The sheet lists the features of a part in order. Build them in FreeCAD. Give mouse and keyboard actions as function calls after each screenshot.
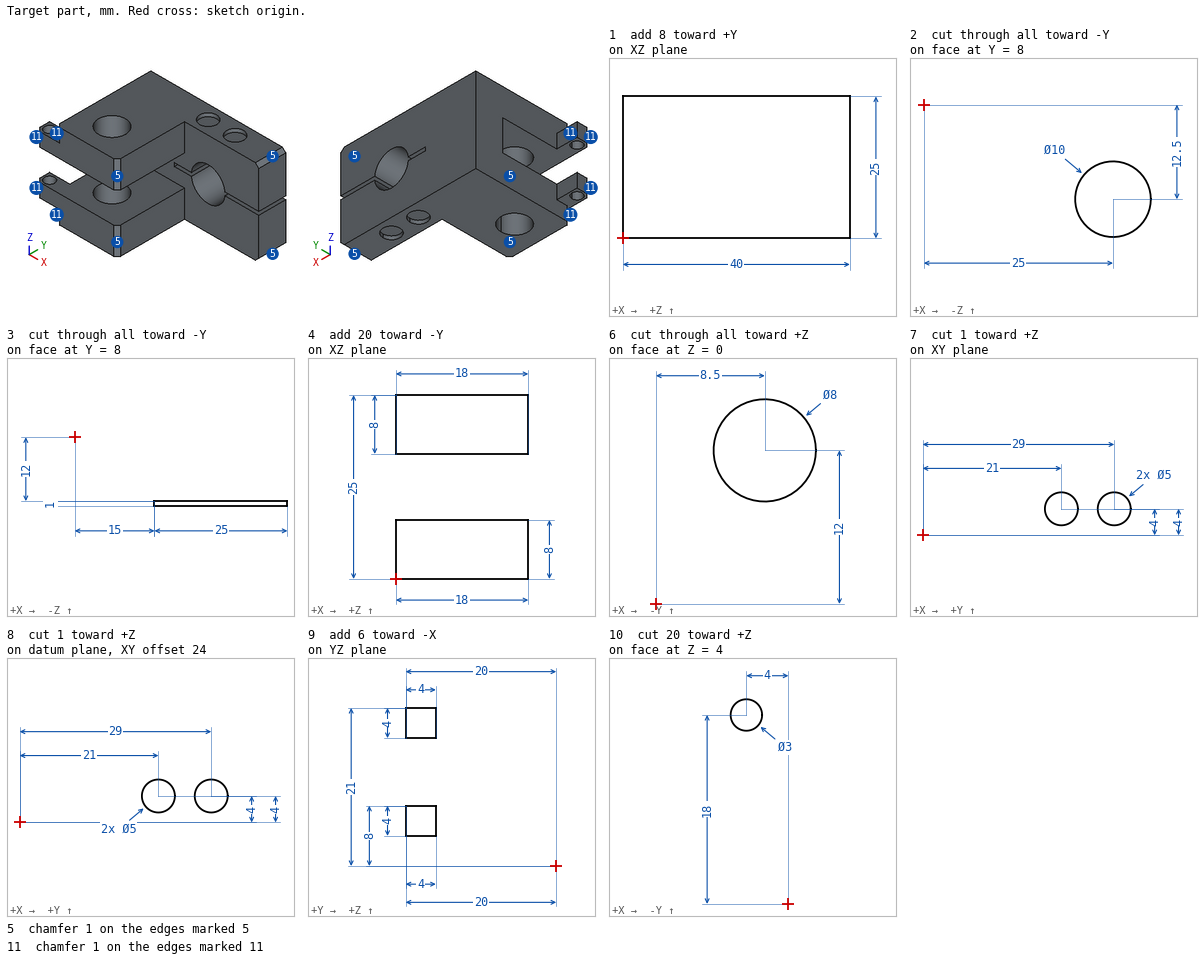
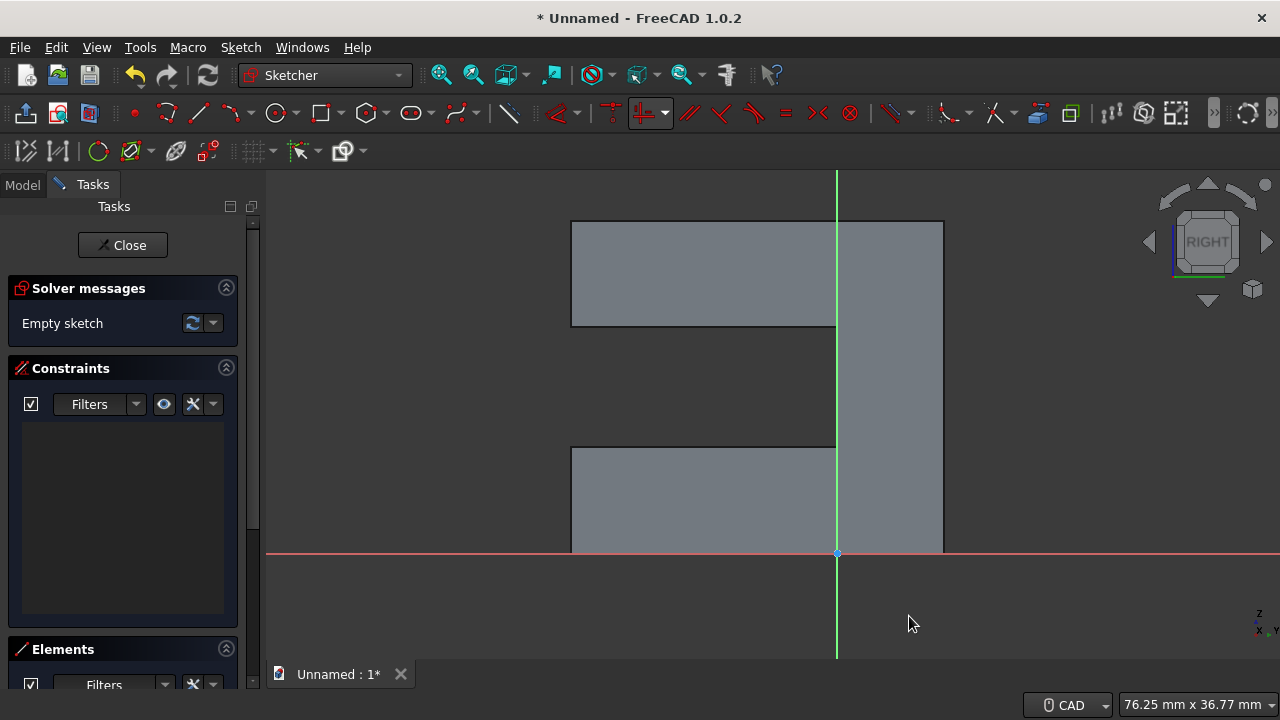
click(322, 114)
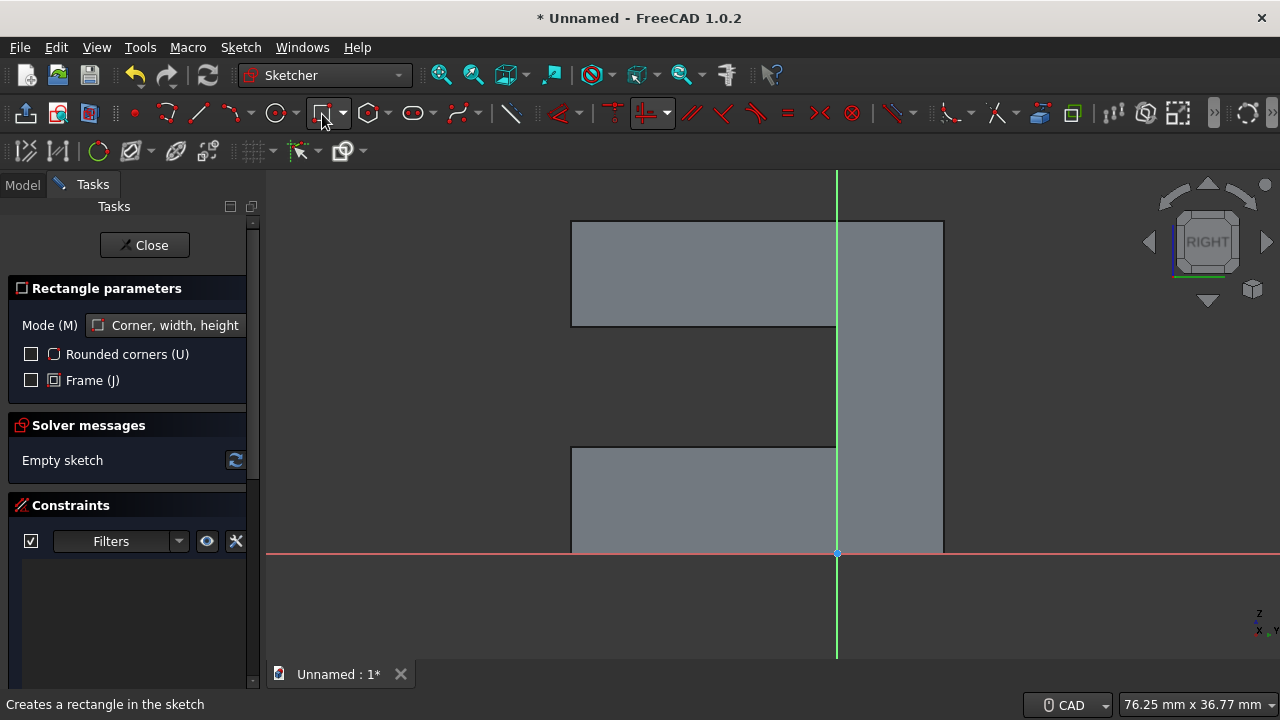
click(571, 274)
click(624, 327)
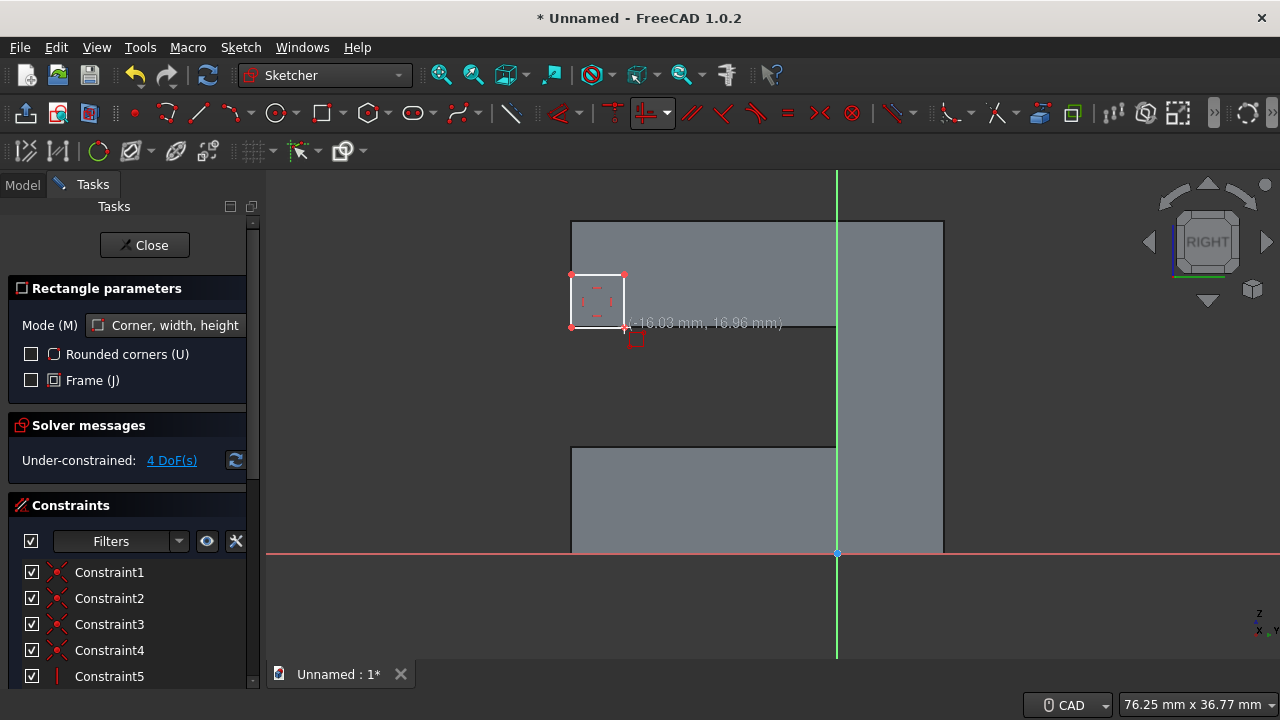
click(571, 447)
click(624, 500)
key(Escape)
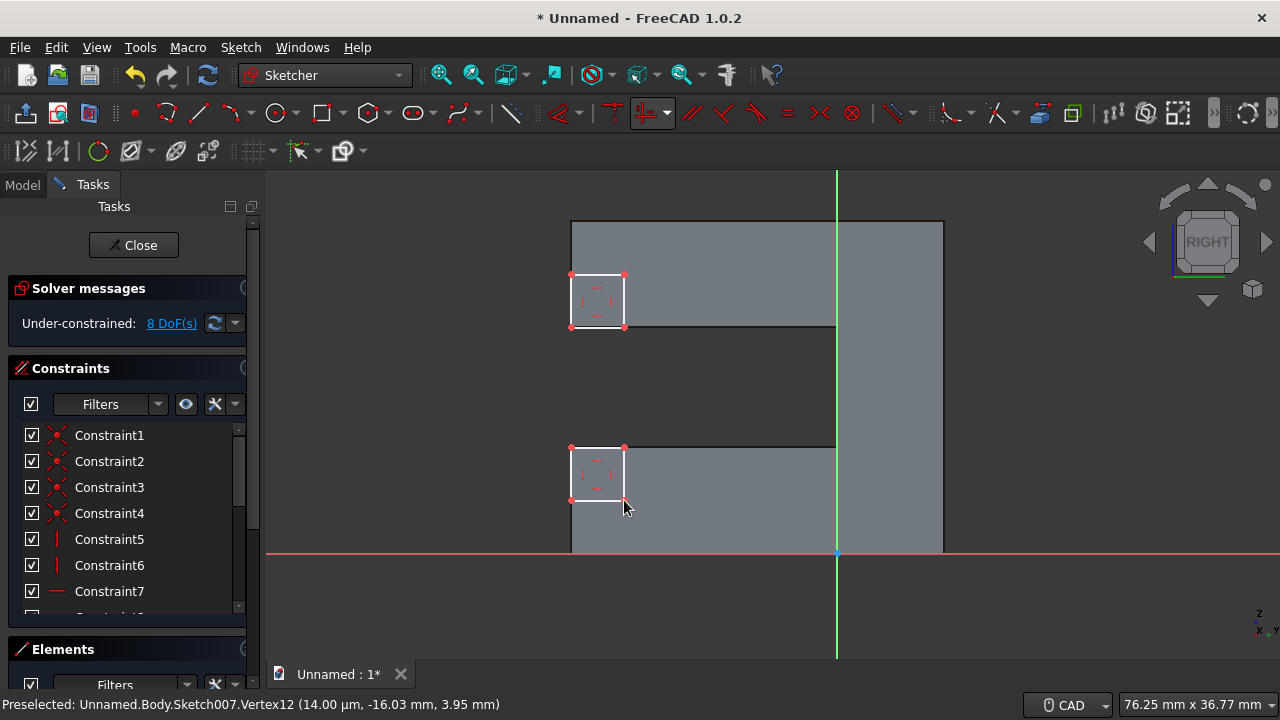
click(558, 114)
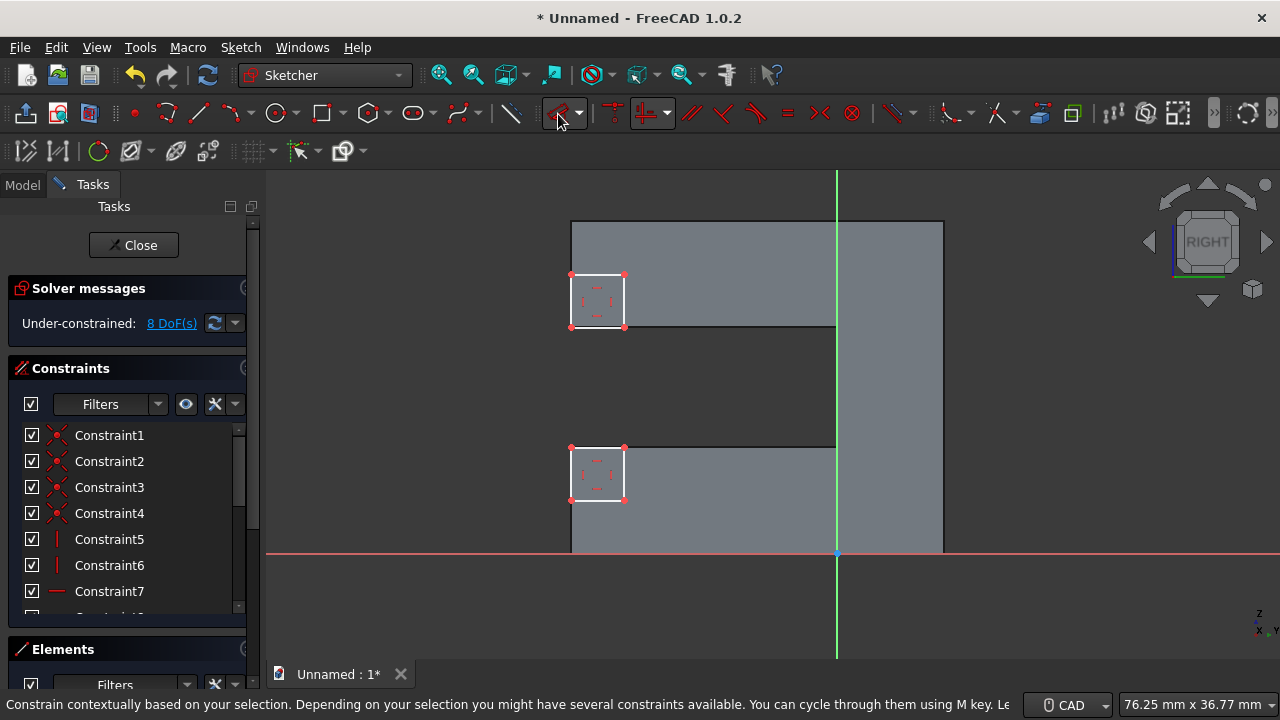
click(571, 291)
click(537, 302)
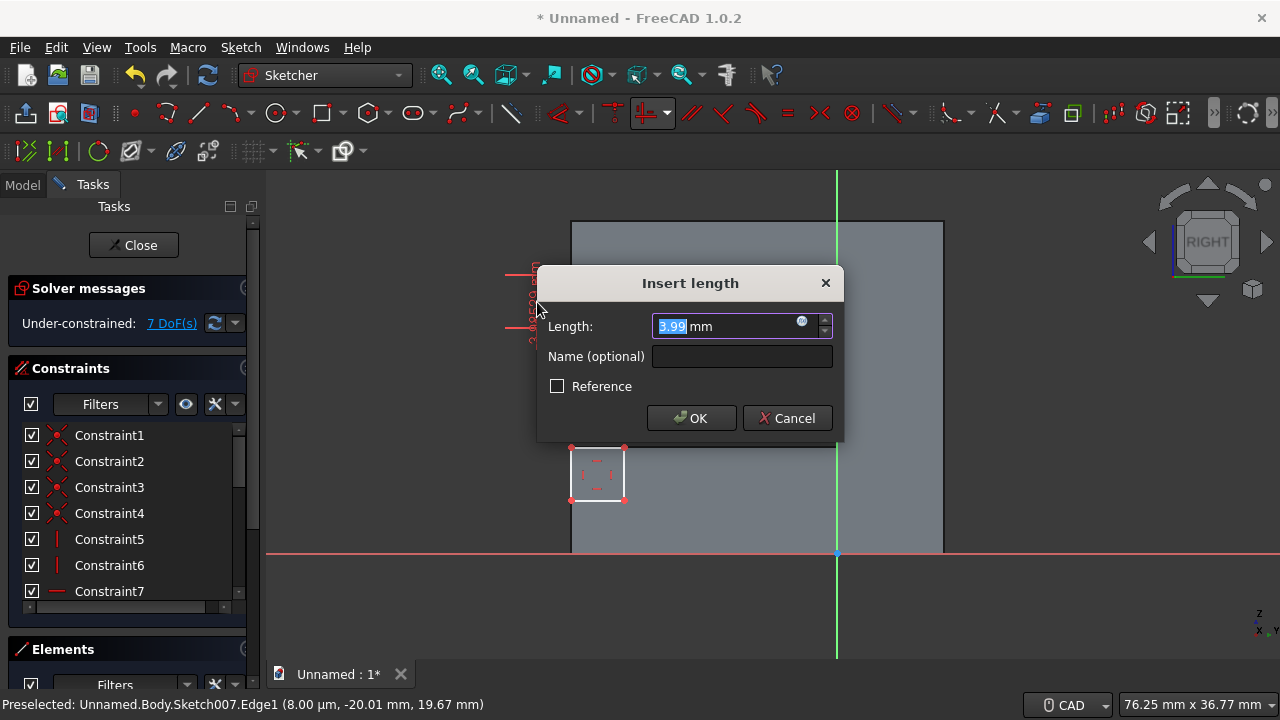
text(4)
key(Return)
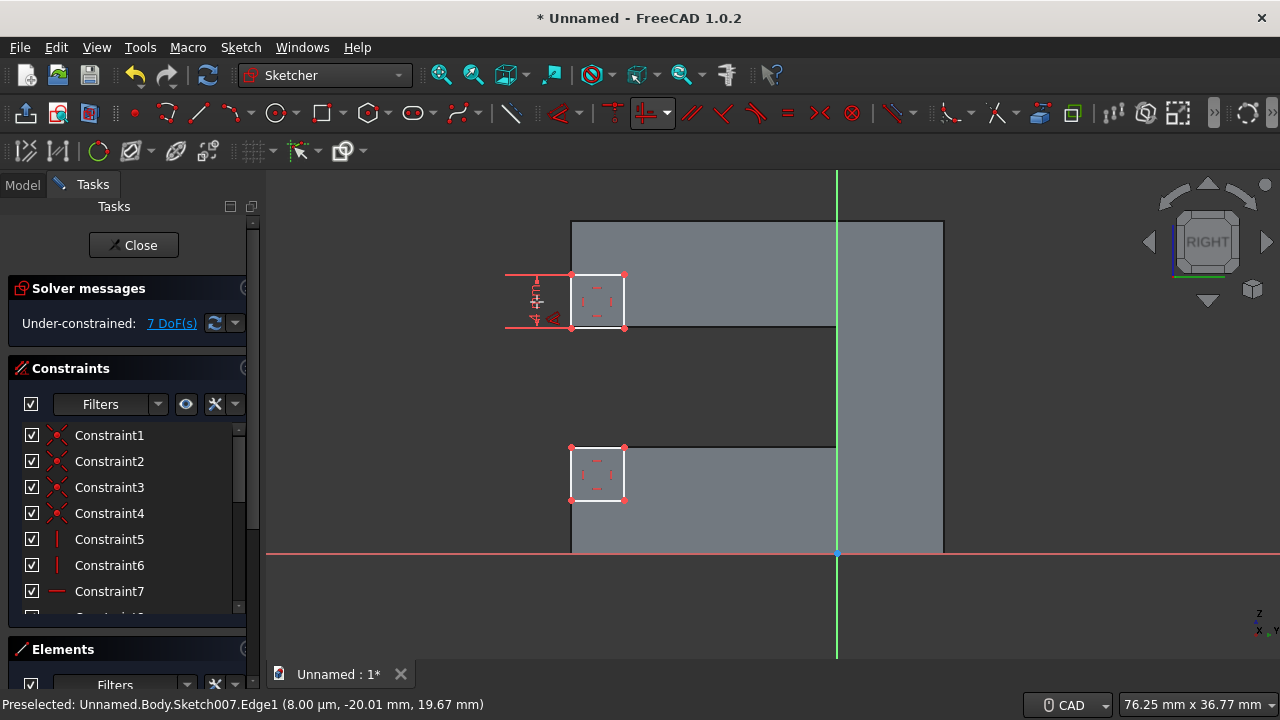
click(587, 328)
click(610, 294)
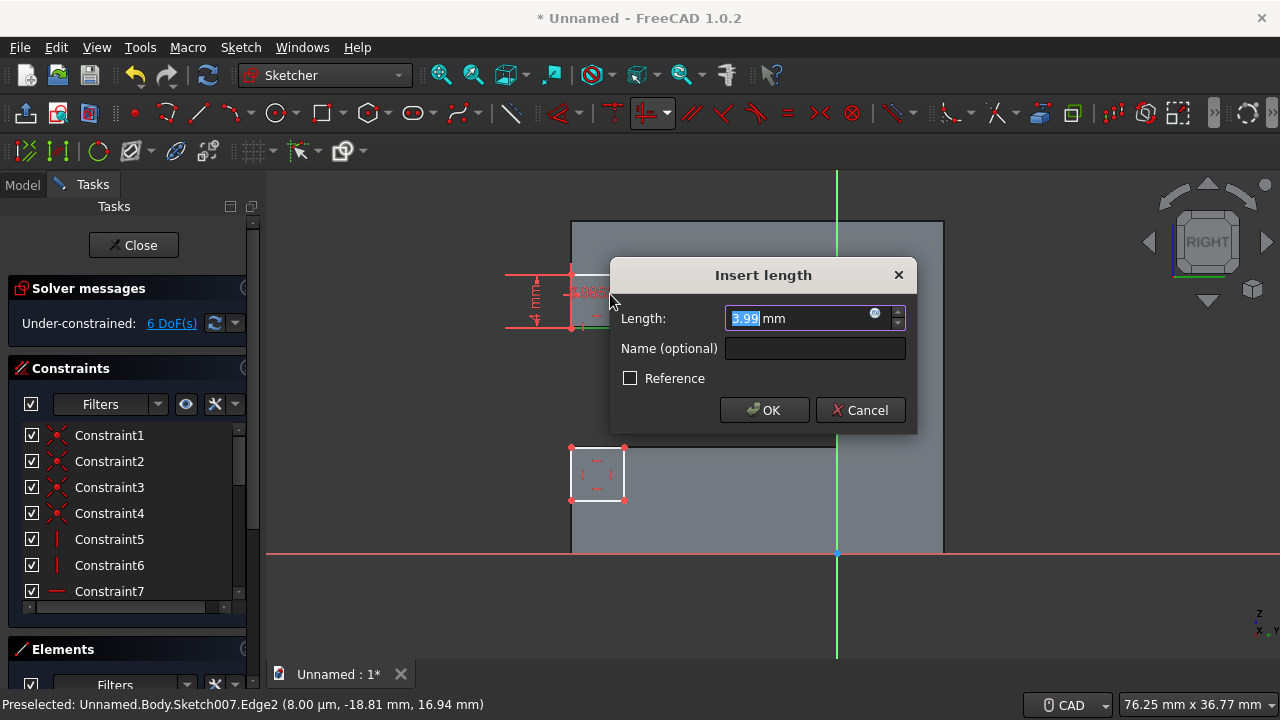
text(4)
key(Return)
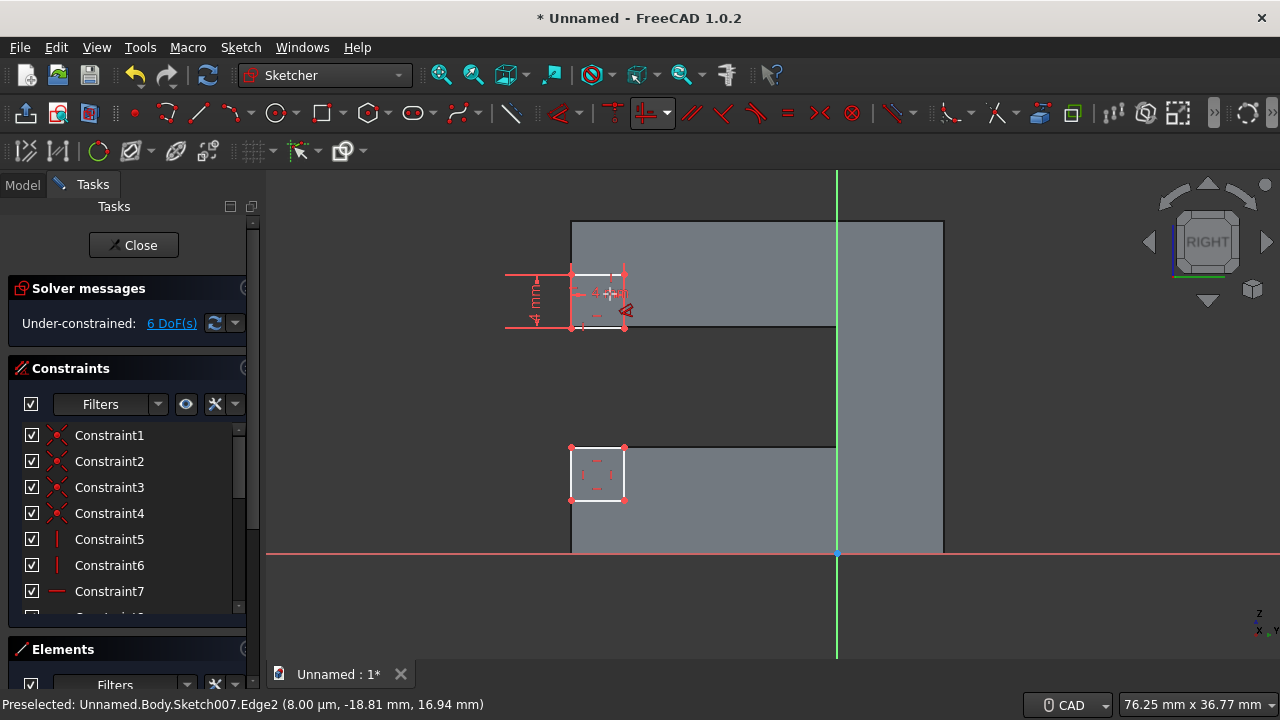
click(571, 464)
click(537, 475)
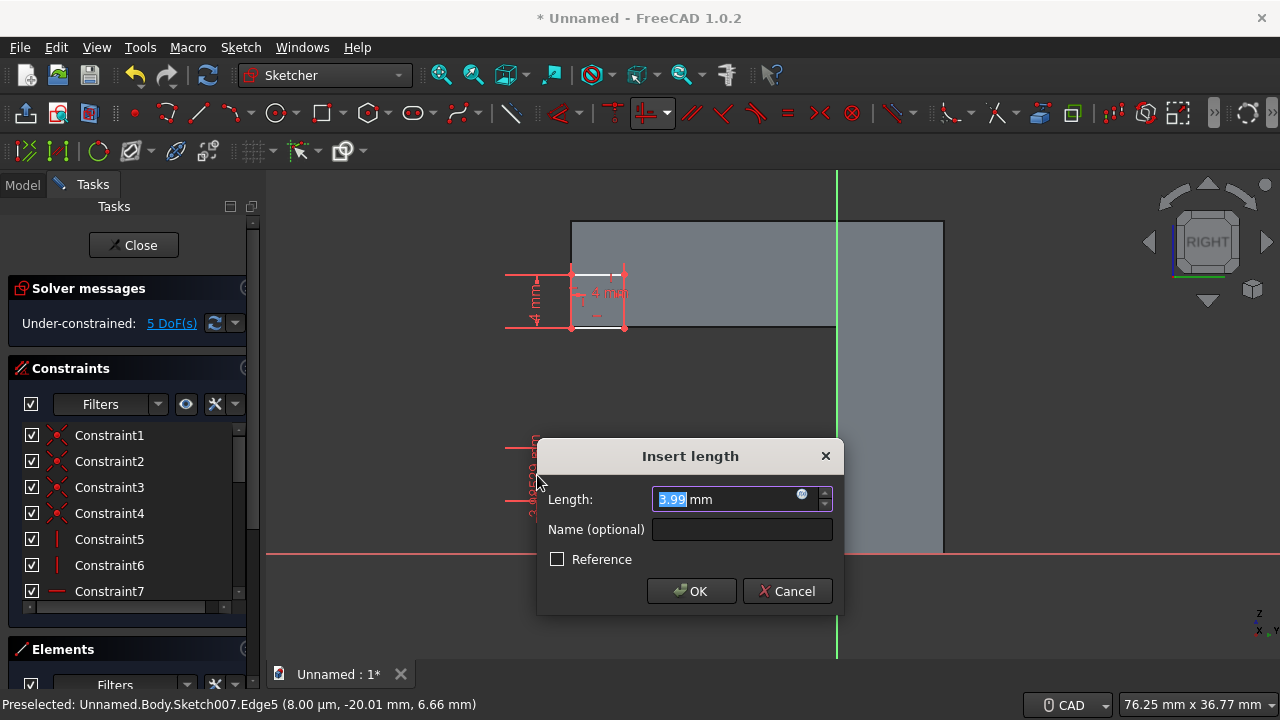
text(4)
key(Return)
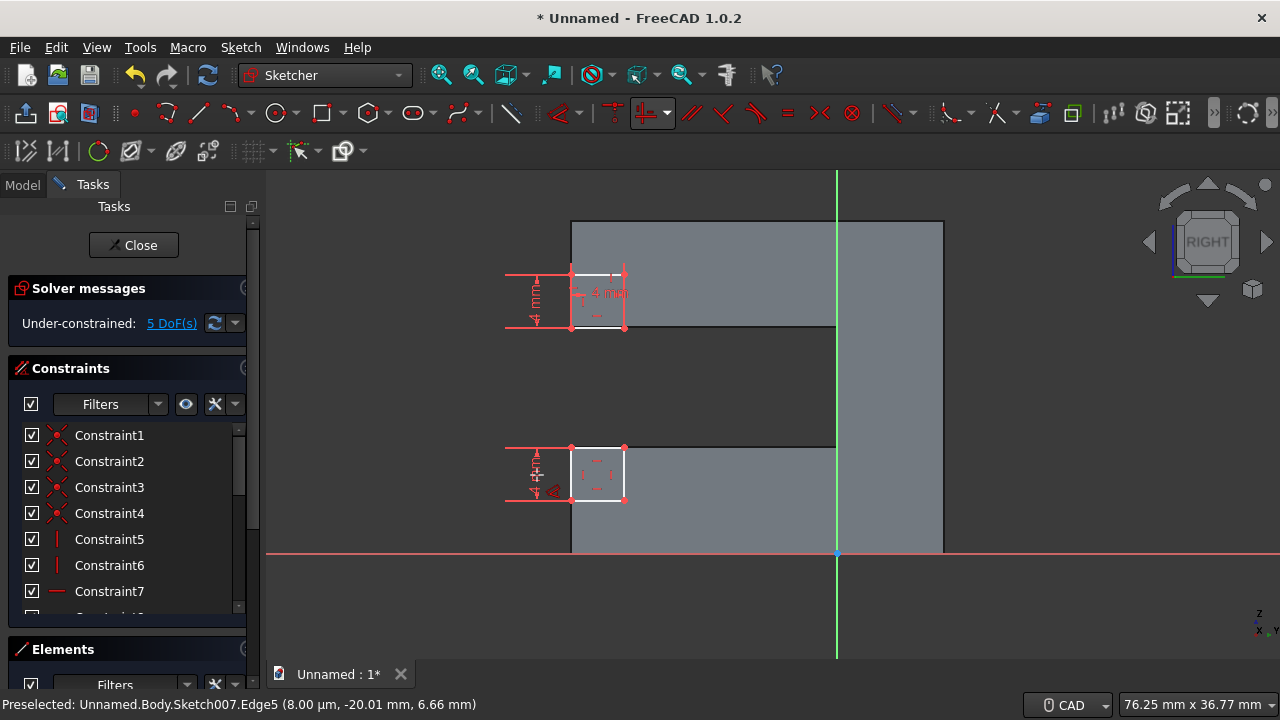
click(587, 501)
click(598, 535)